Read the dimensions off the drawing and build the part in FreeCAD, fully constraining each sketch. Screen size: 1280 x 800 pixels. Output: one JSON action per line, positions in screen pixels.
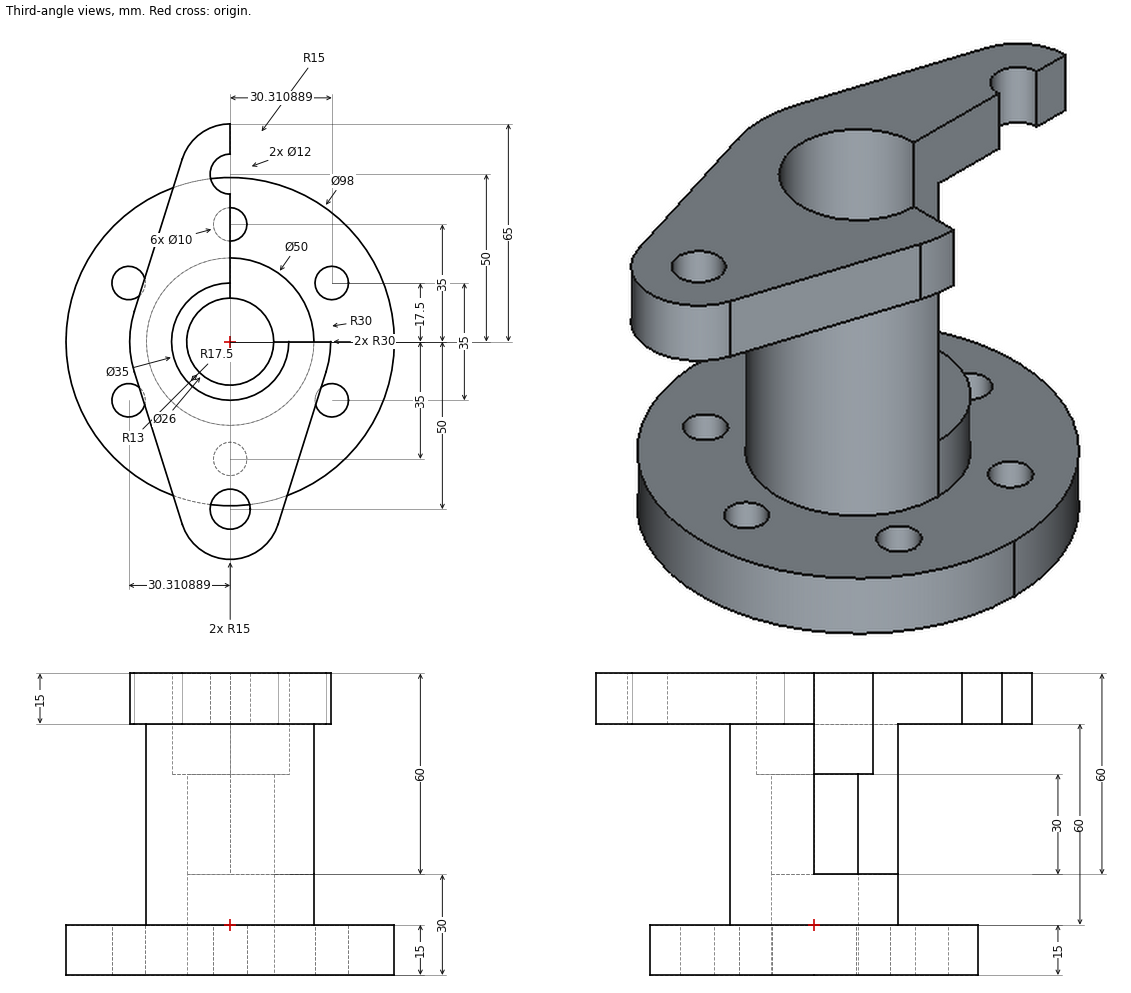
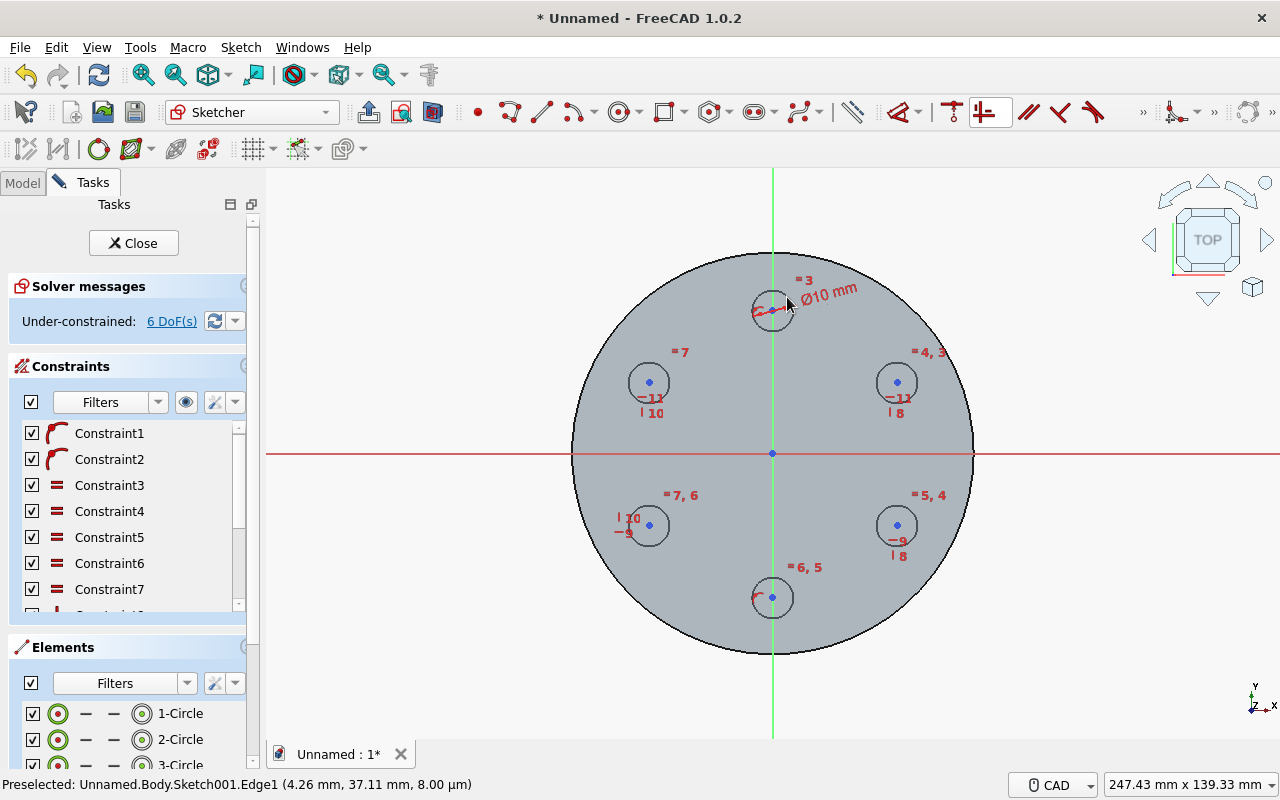
{"action": "left_click", "coordinate": [773, 311]}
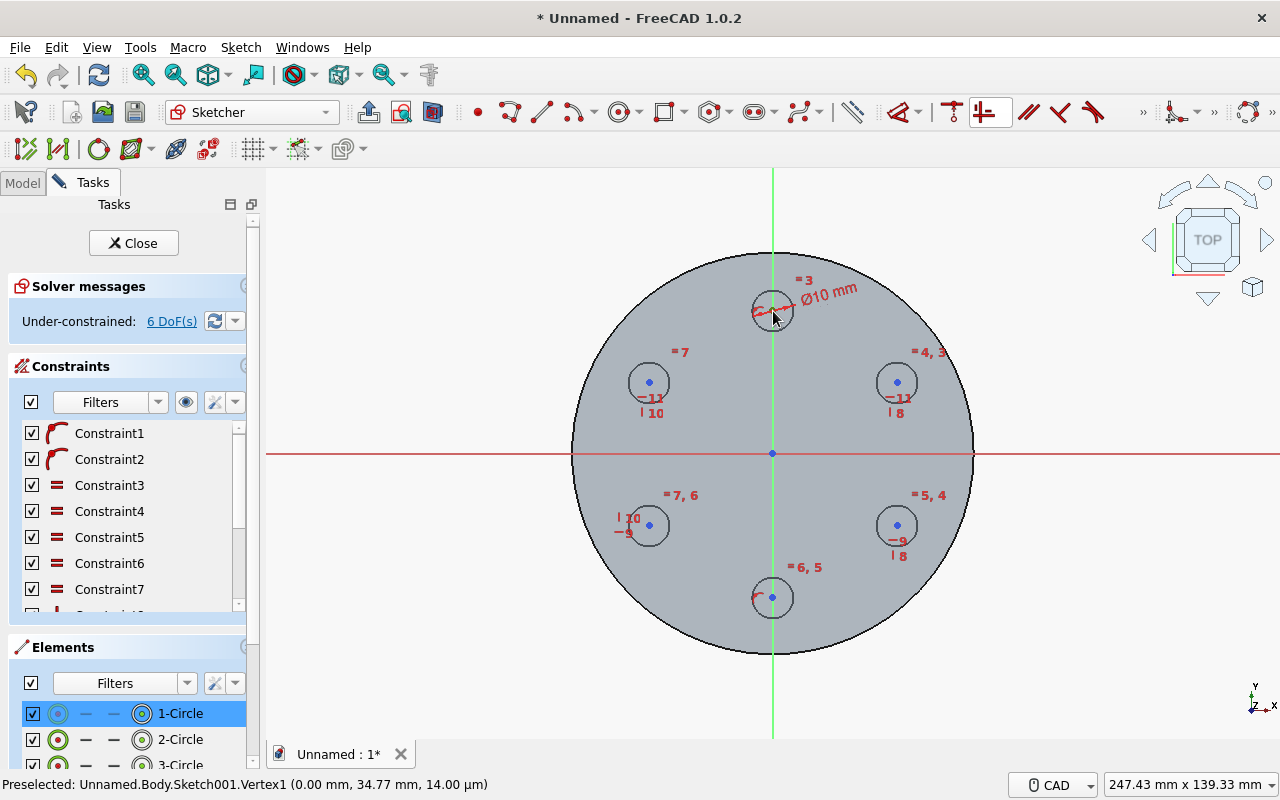
{"action": "key", "text": "i"}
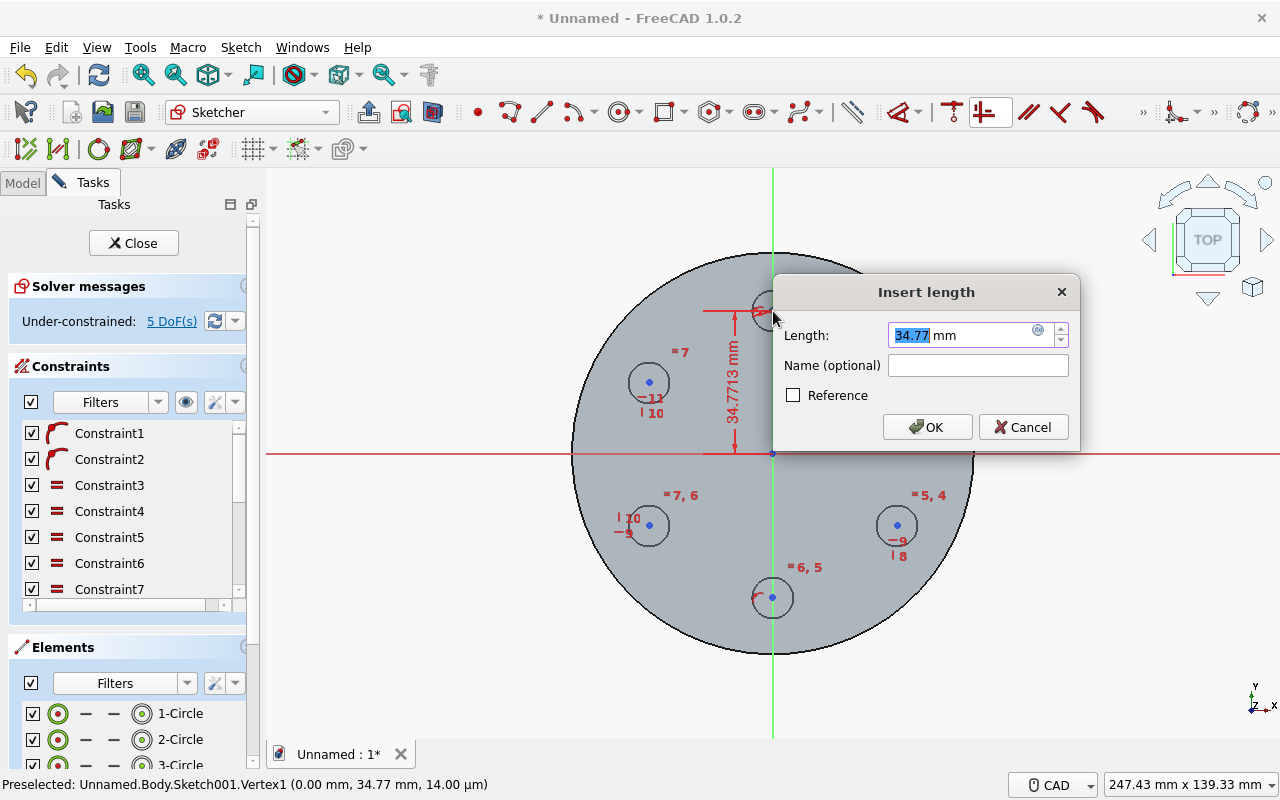
{"action": "type", "text": "35"}
{"action": "key", "text": "Return"}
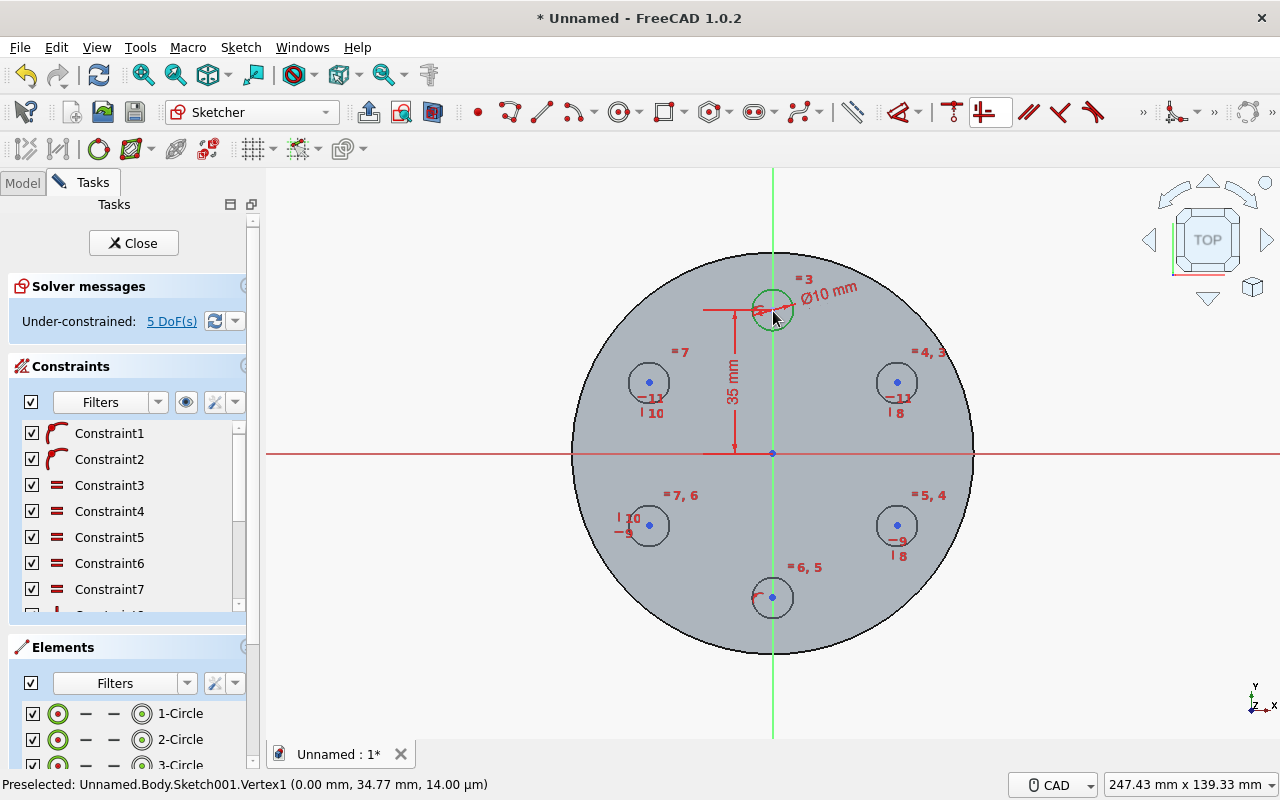
{"action": "left_click", "coordinate": [773, 598]}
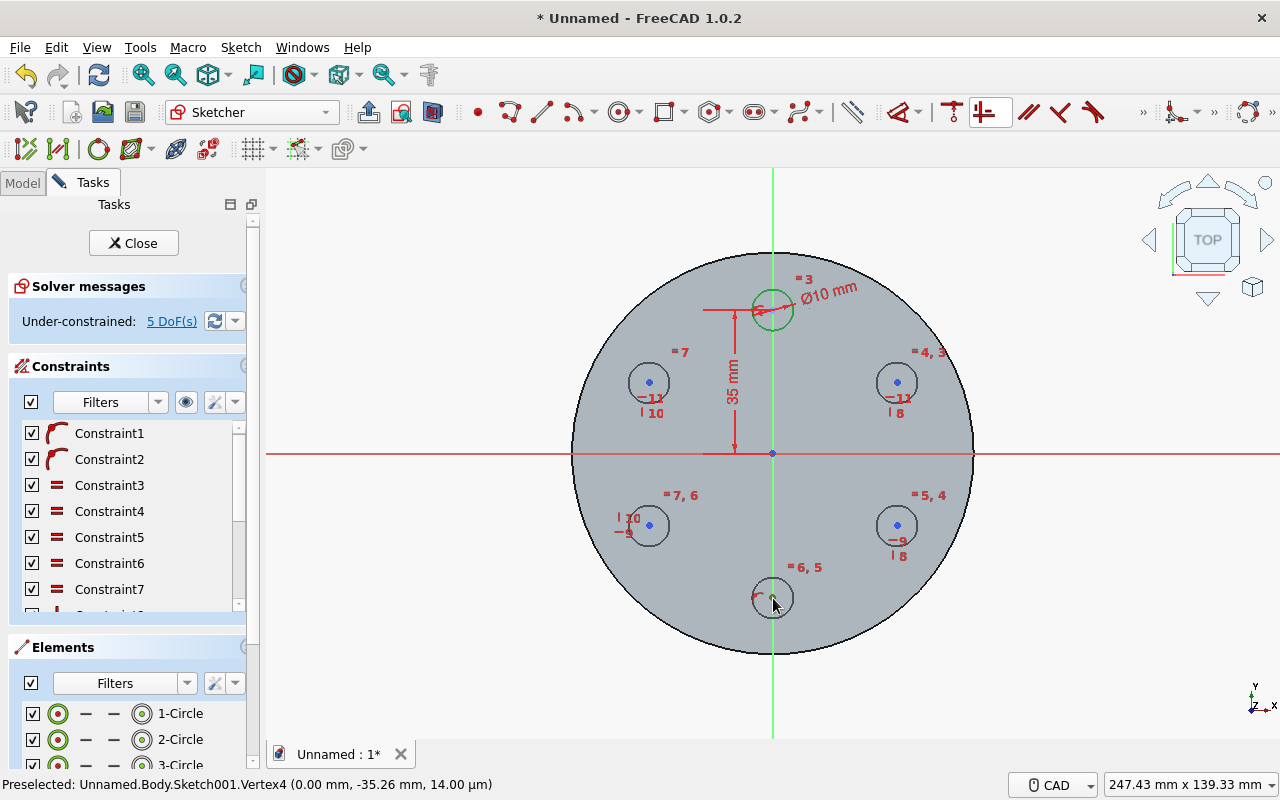
{"action": "key", "text": "i"}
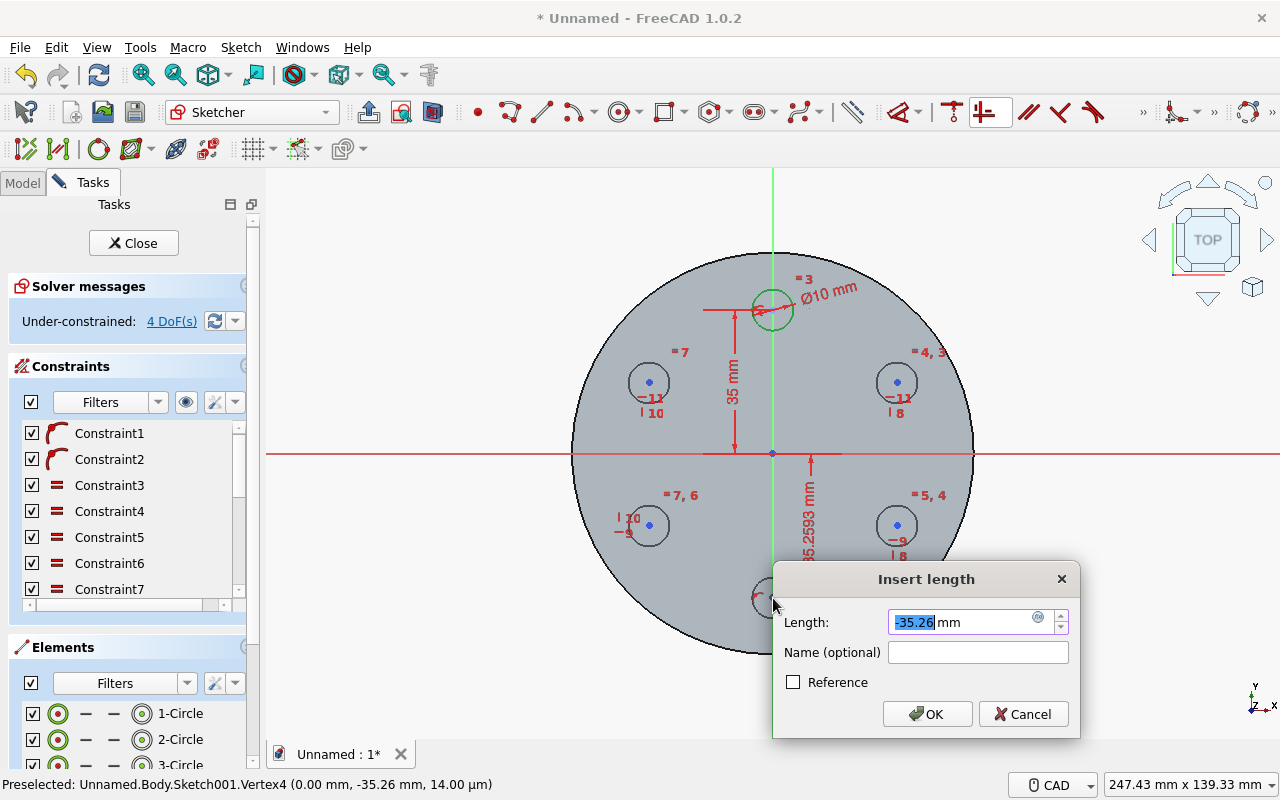
{"action": "type", "text": "-35"}
{"action": "key", "text": "Return"}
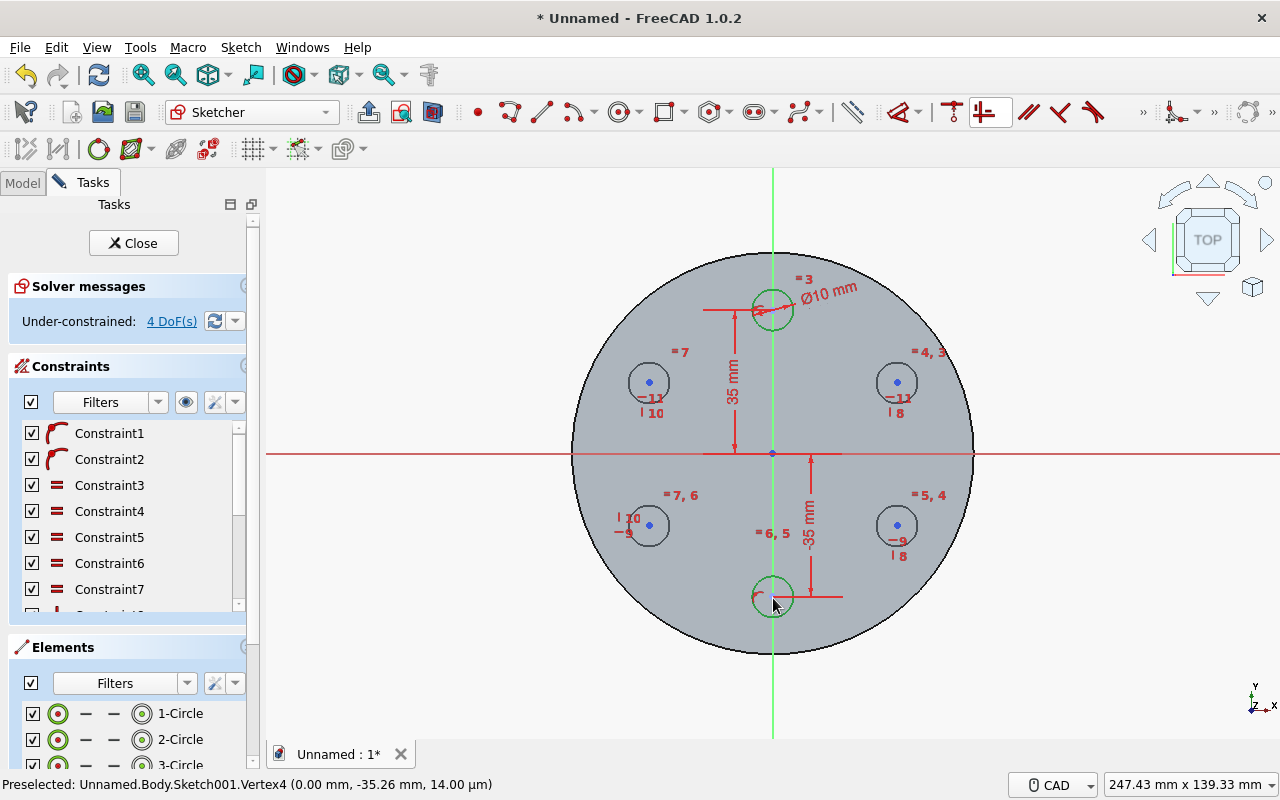
{"action": "left_click", "coordinate": [897, 383]}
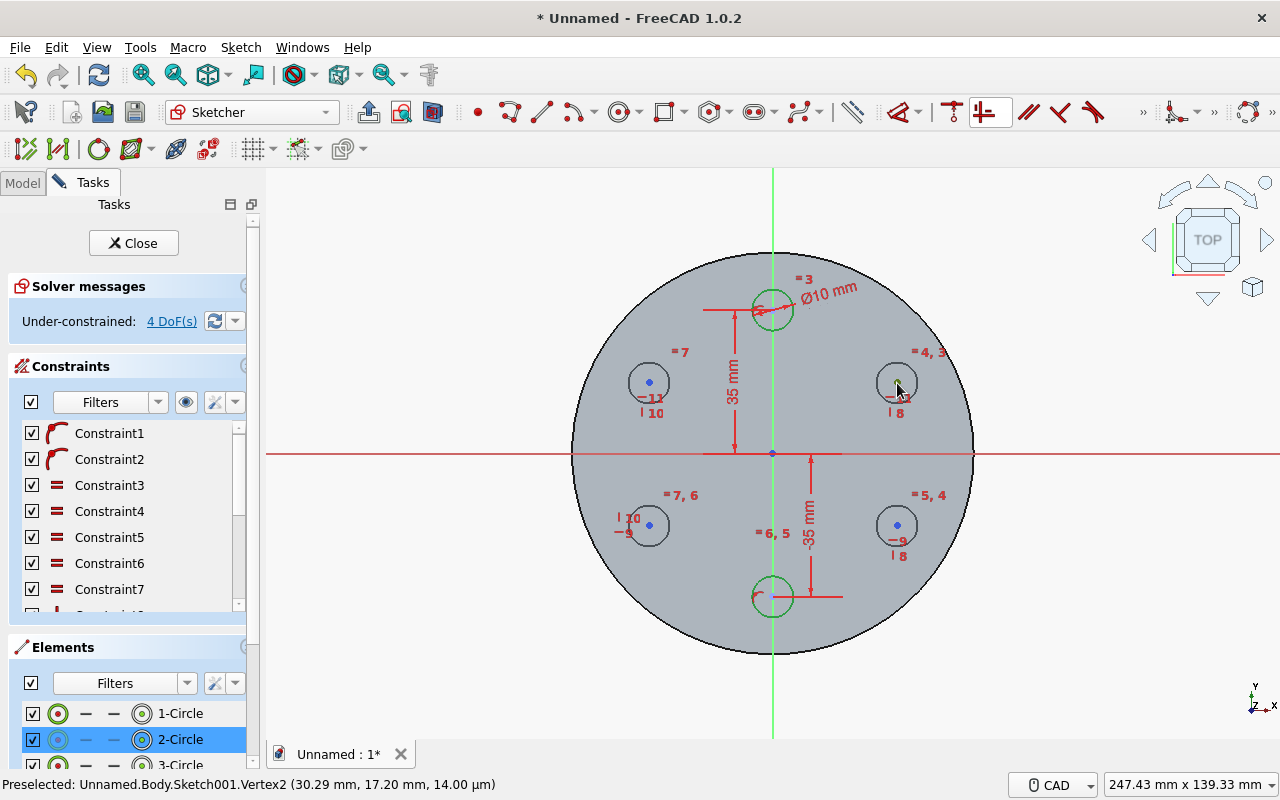
{"action": "left_click", "coordinate": [897, 526]}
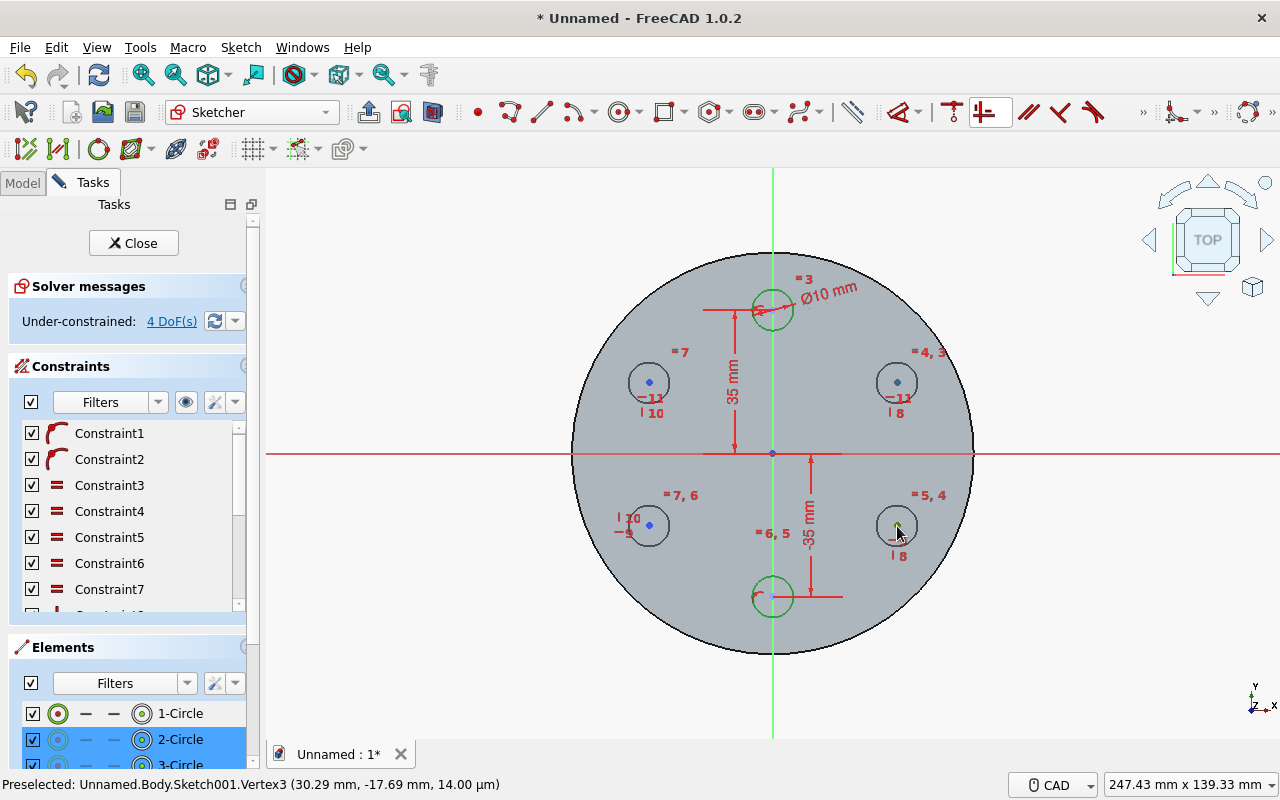
{"action": "key", "text": "i"}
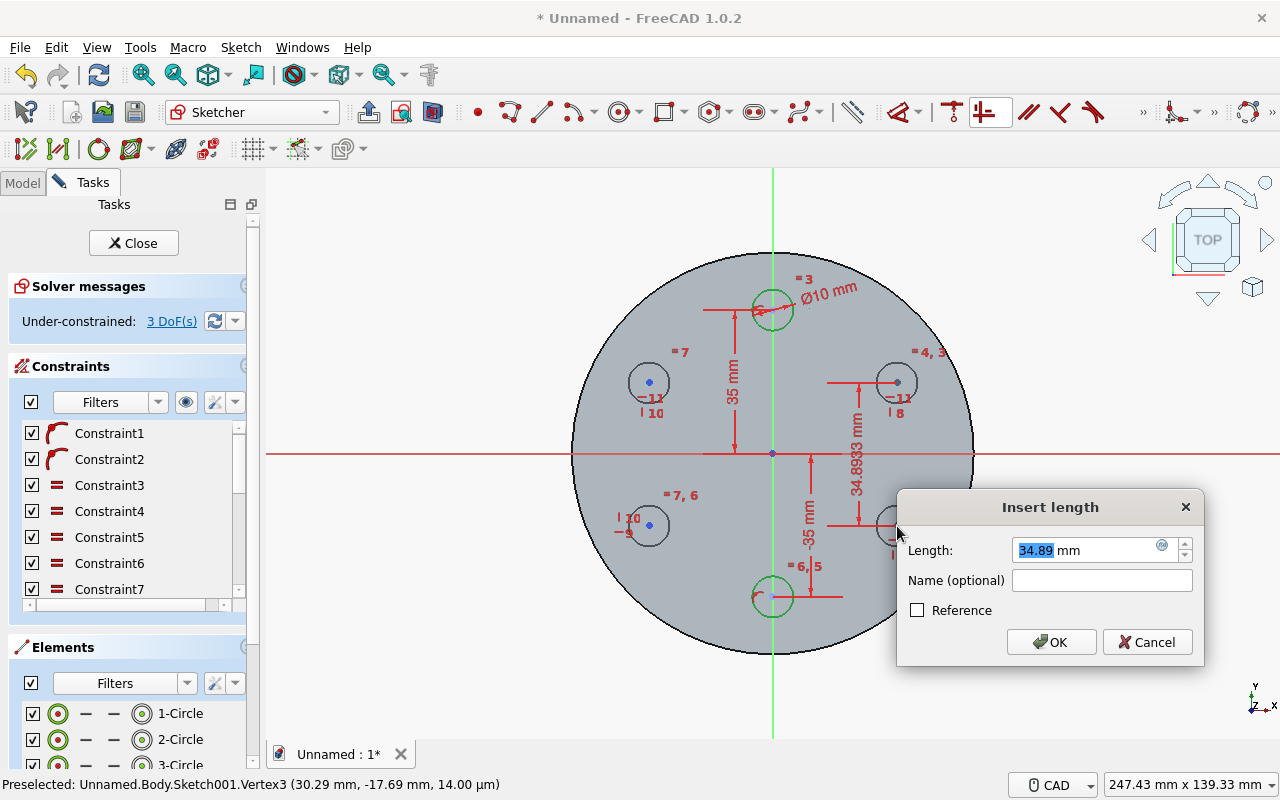
{"action": "type", "text": "35"}
{"action": "key", "text": "Return"}